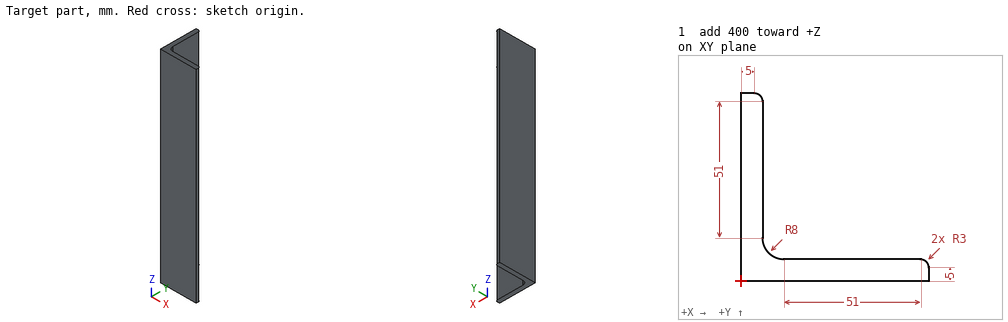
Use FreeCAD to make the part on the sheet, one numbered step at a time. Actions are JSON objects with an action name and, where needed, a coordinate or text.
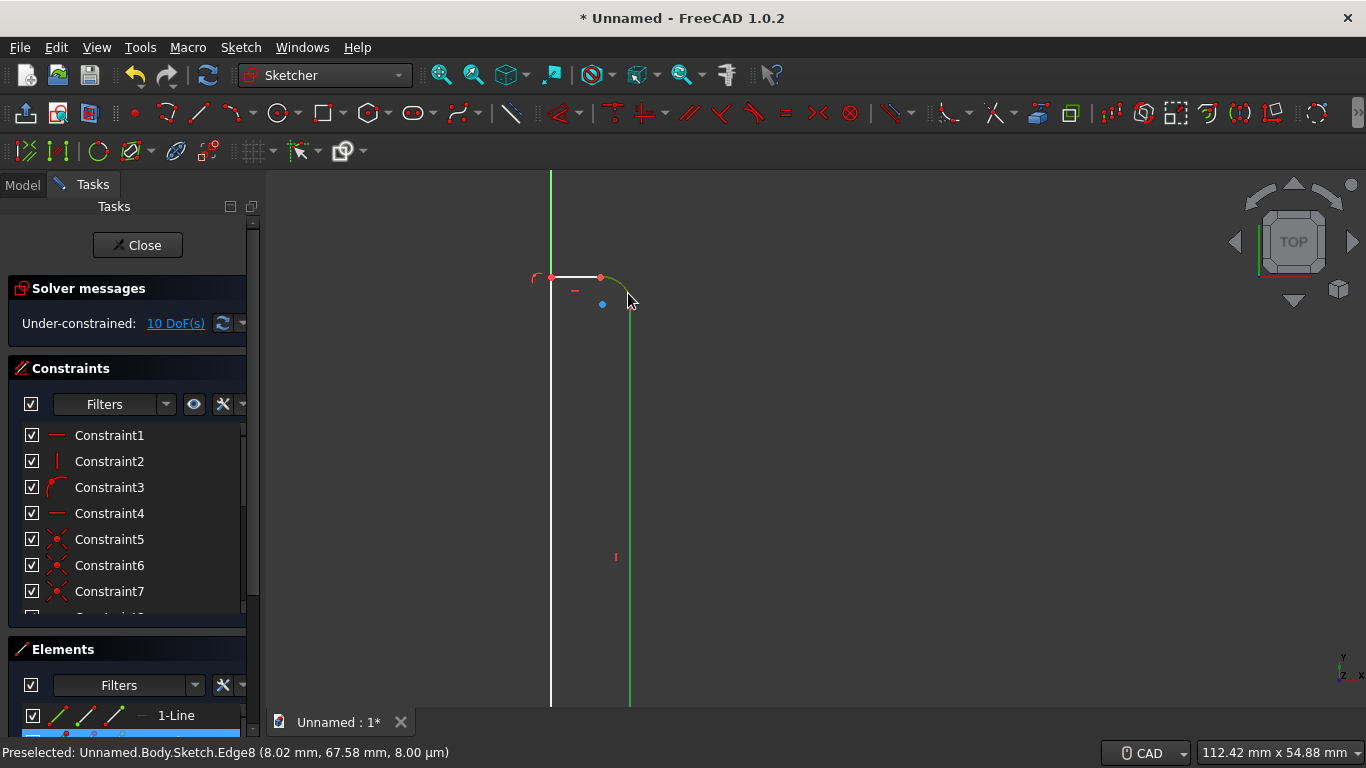
{"action": "left_click", "coordinate": [754, 114]}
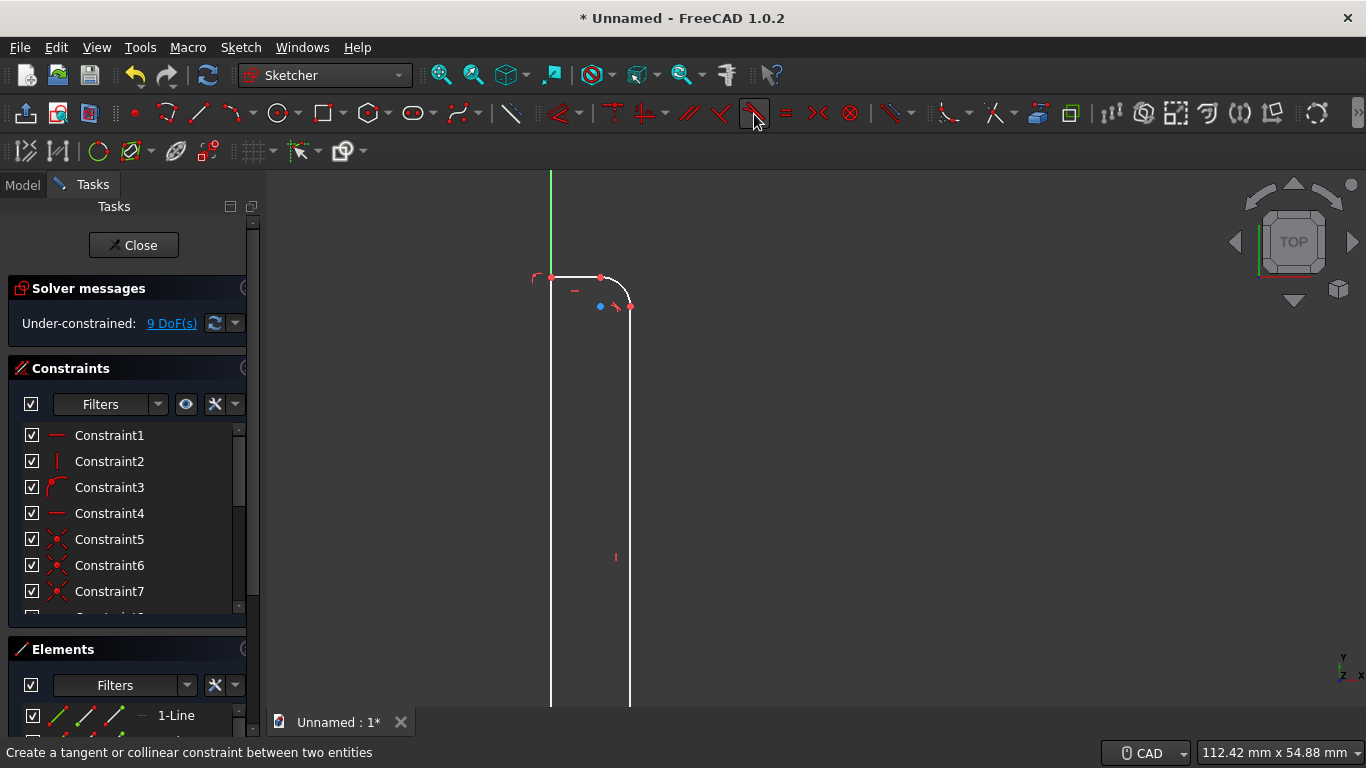
{"action": "left_click", "coordinate": [586, 277]}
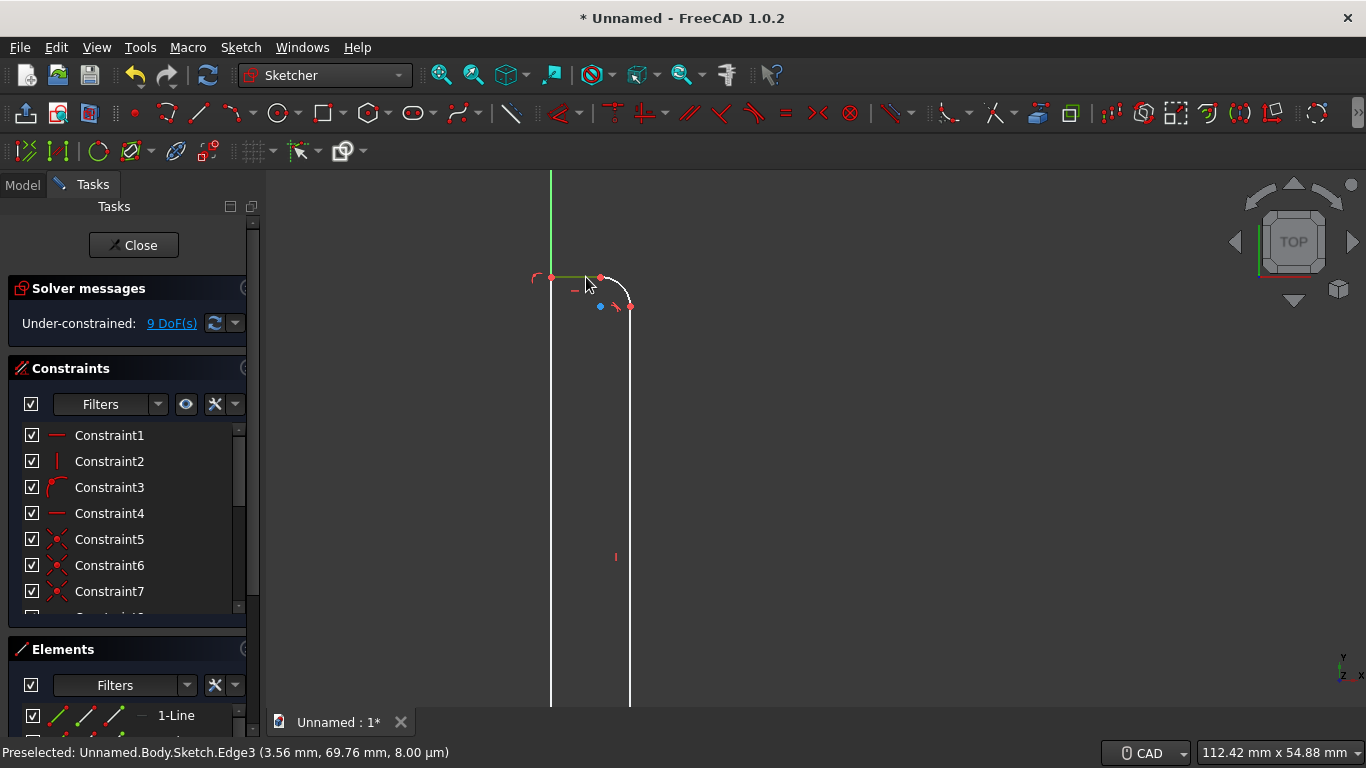
{"action": "left_click", "coordinate": [627, 293]}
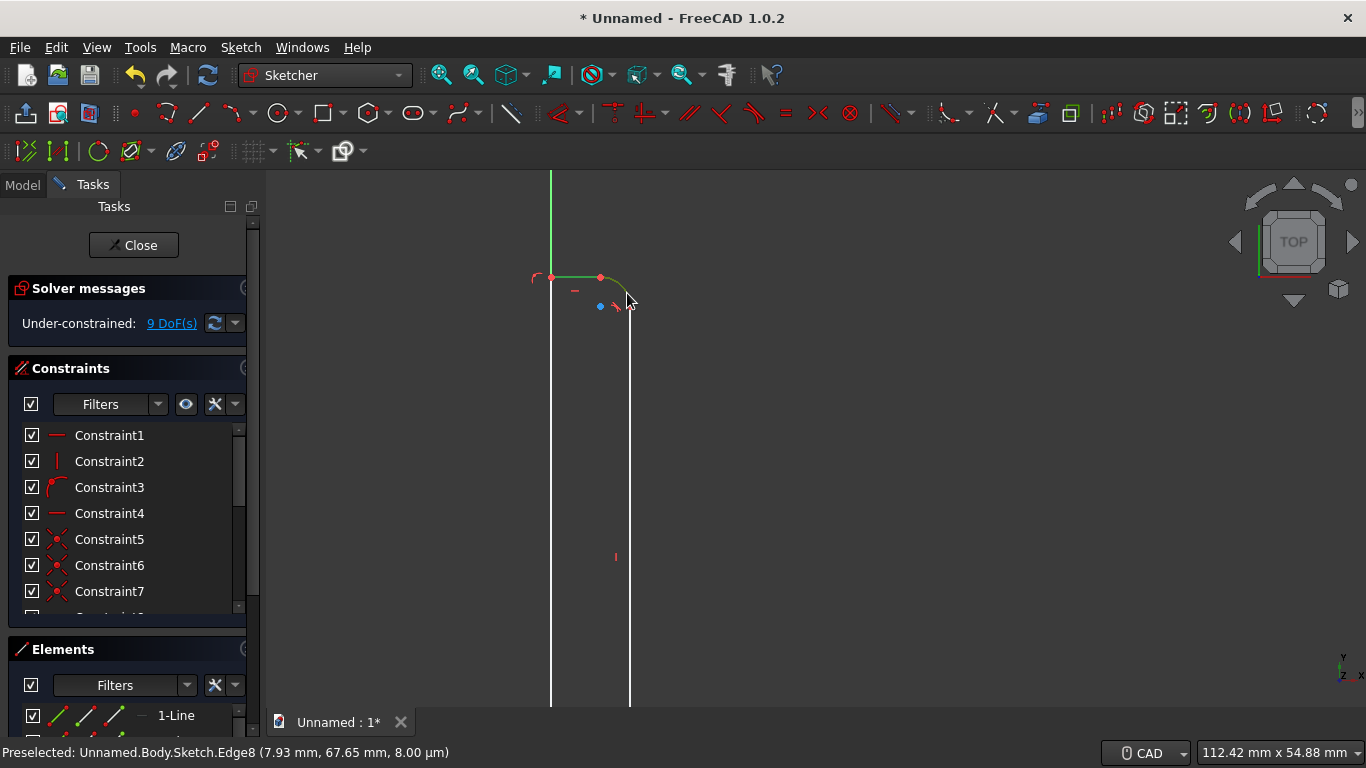
{"action": "left_click", "coordinate": [754, 114]}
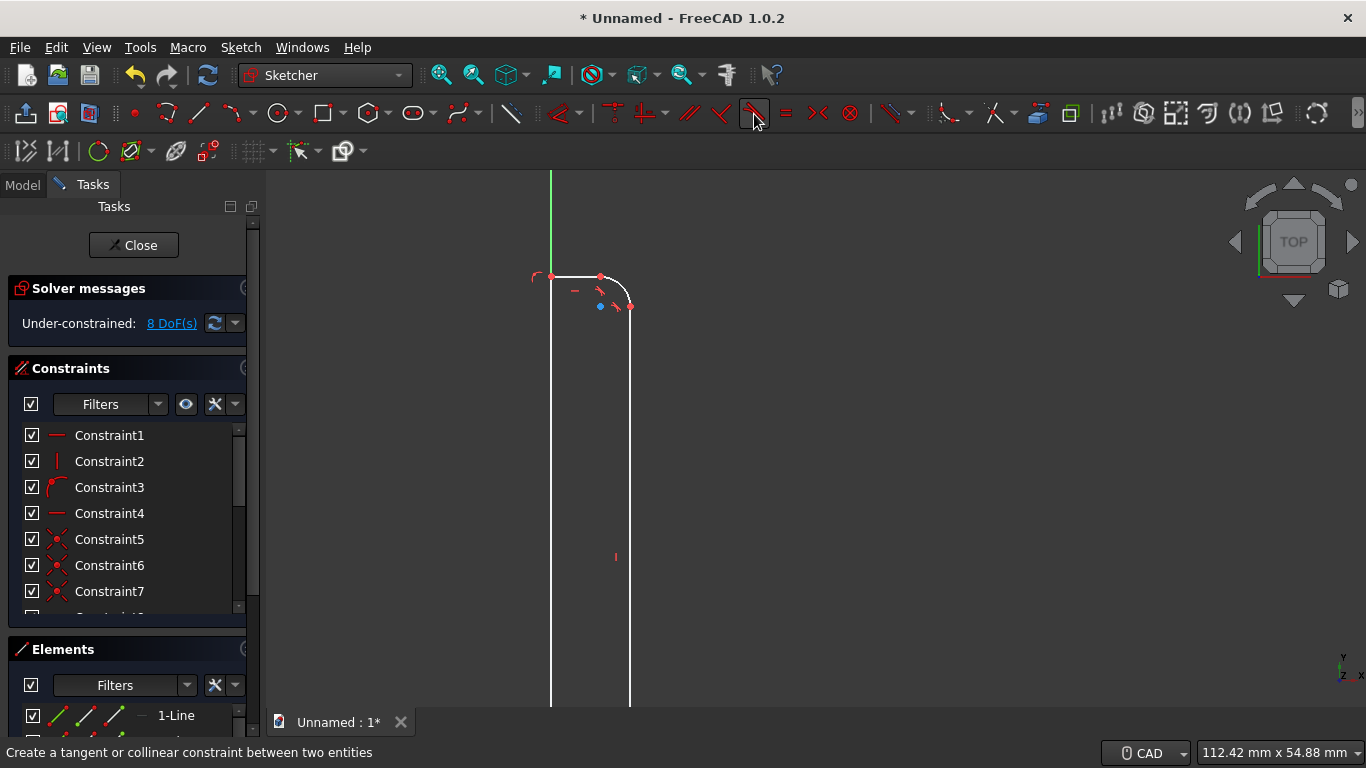
{"action": "scroll", "coordinate": [628, 293], "scroll_direction": "down", "scroll_amount": 4}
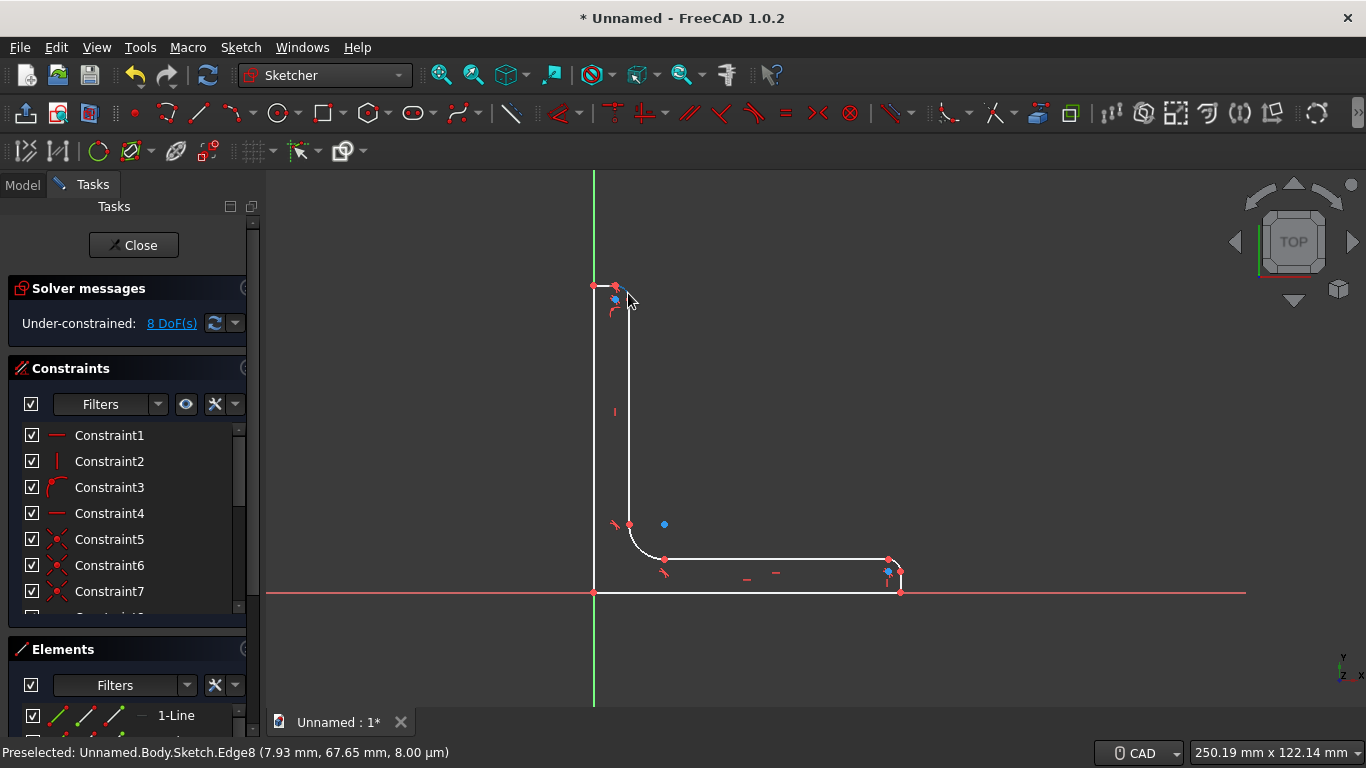
{"action": "scroll", "coordinate": [901, 586], "scroll_direction": "up", "scroll_amount": 4}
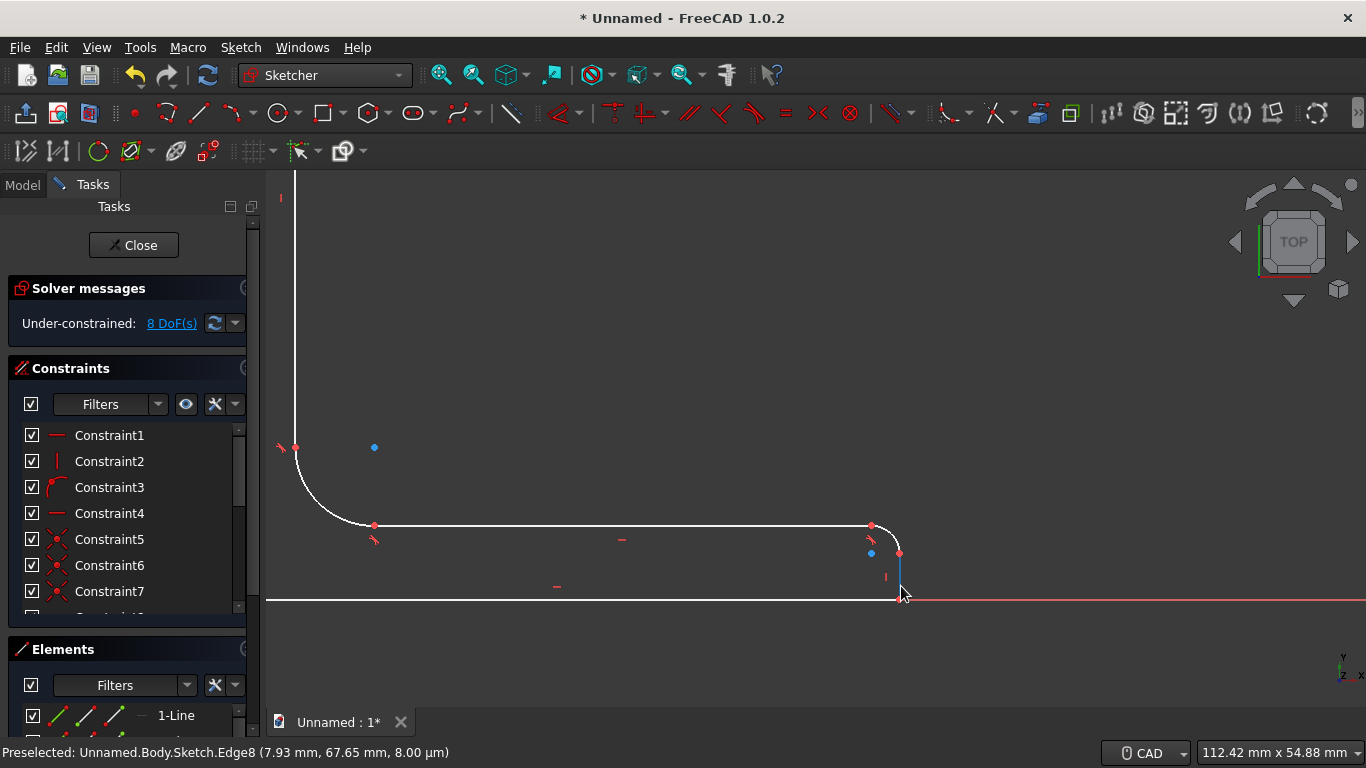
{"action": "left_click", "coordinate": [900, 586]}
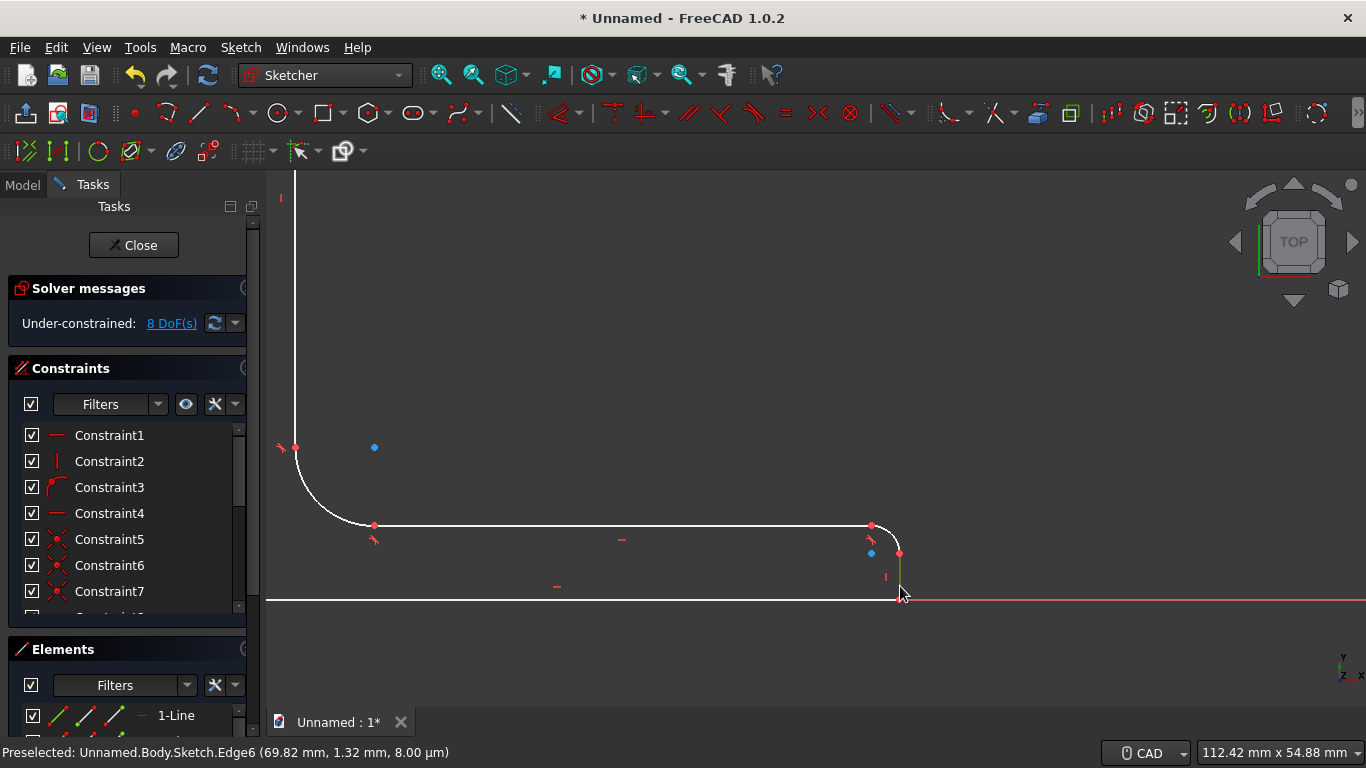
{"action": "left_click", "coordinate": [896, 541]}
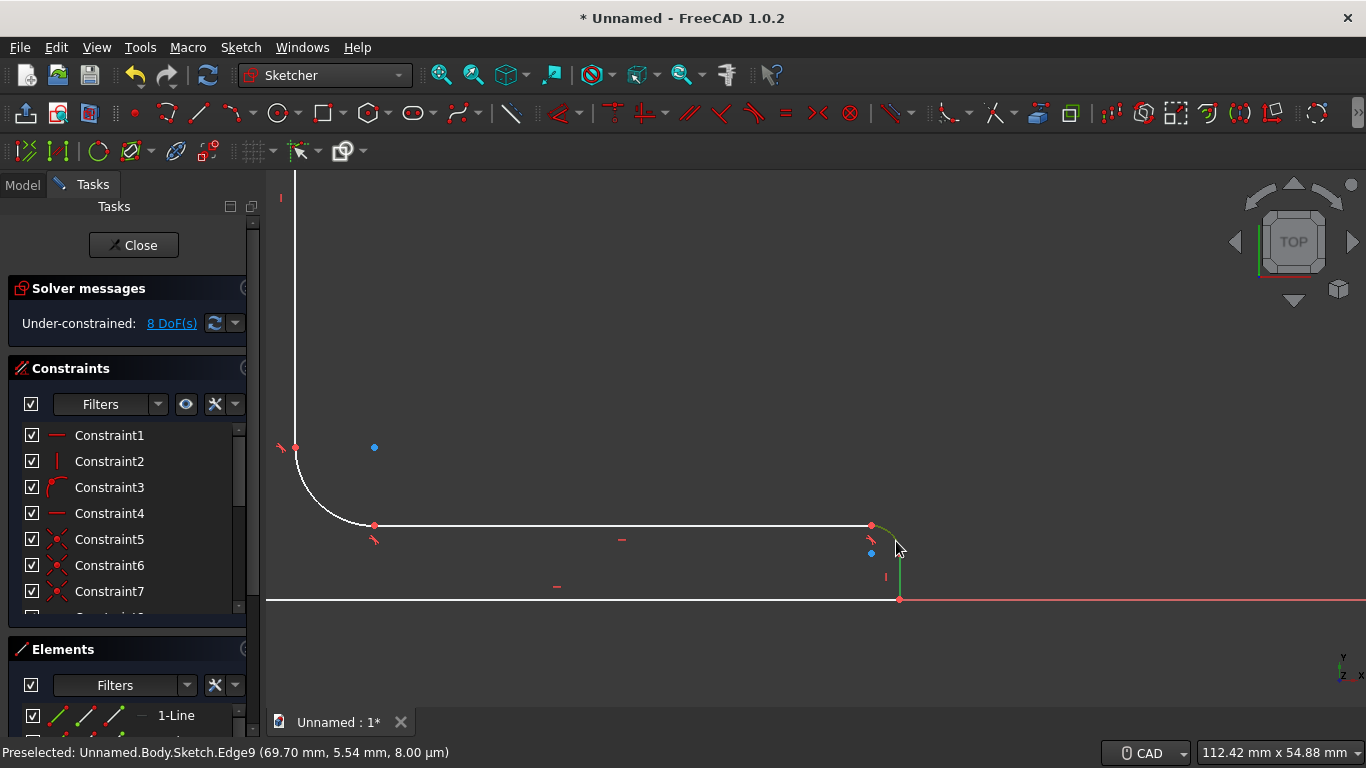
{"action": "left_click", "coordinate": [754, 114]}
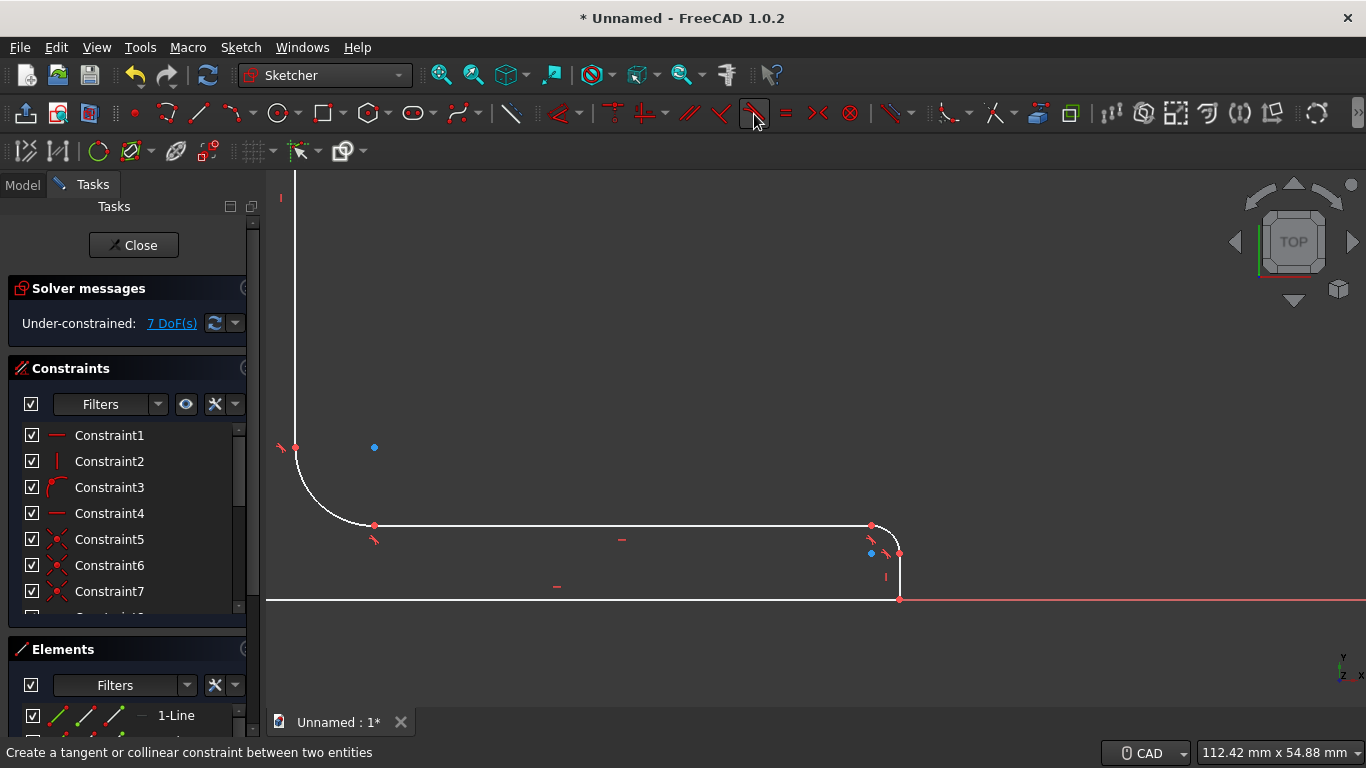
{"action": "scroll", "coordinate": [901, 586], "scroll_direction": "down", "scroll_amount": 4}